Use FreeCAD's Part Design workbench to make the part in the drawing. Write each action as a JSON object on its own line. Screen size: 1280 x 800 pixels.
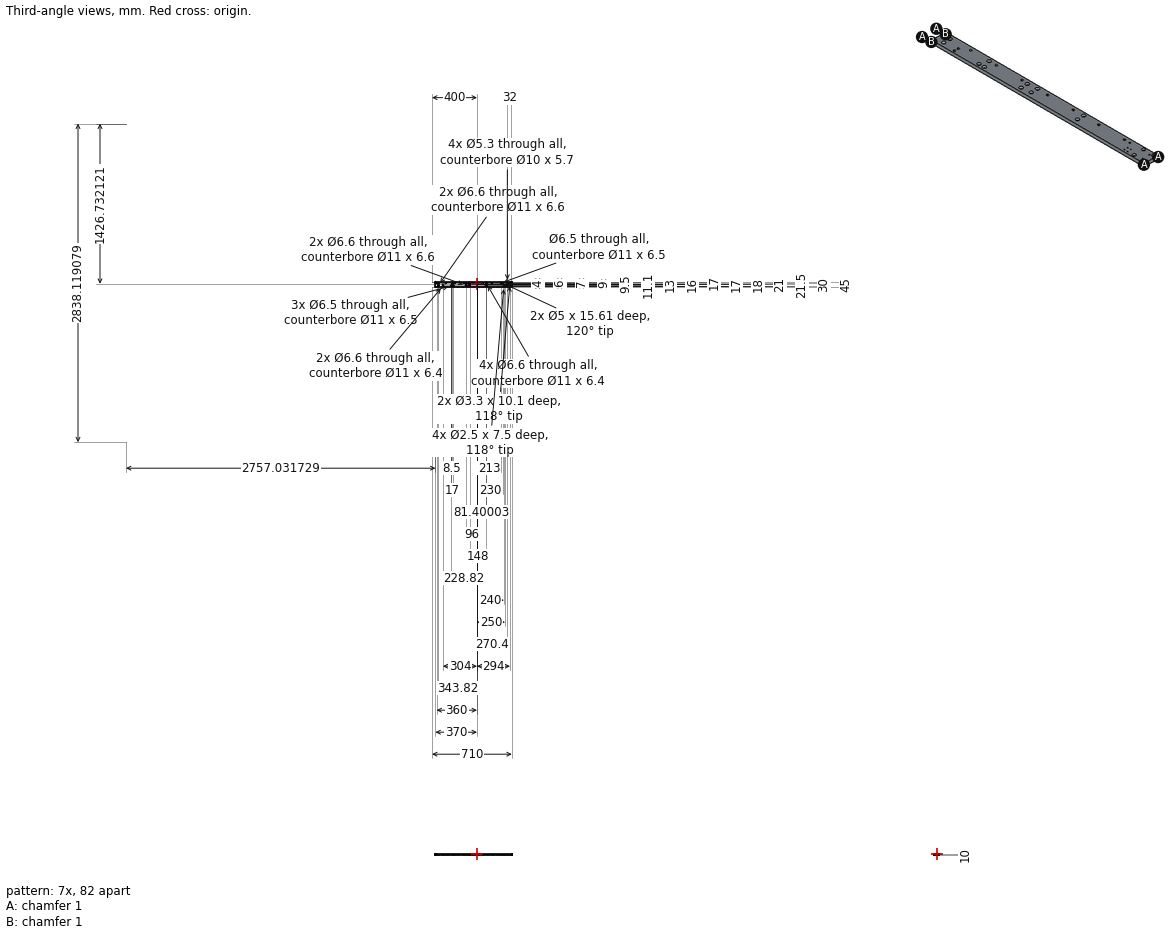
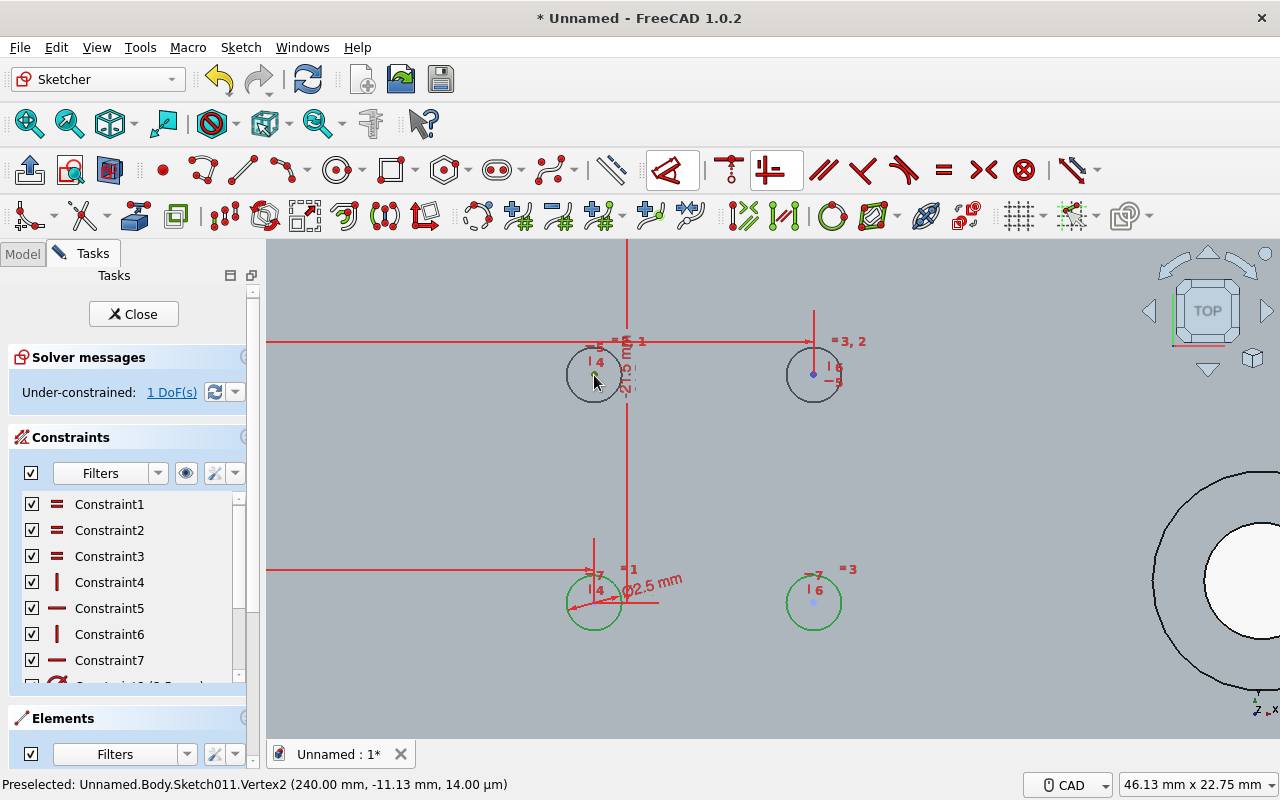
{"action": "key", "text": "i"}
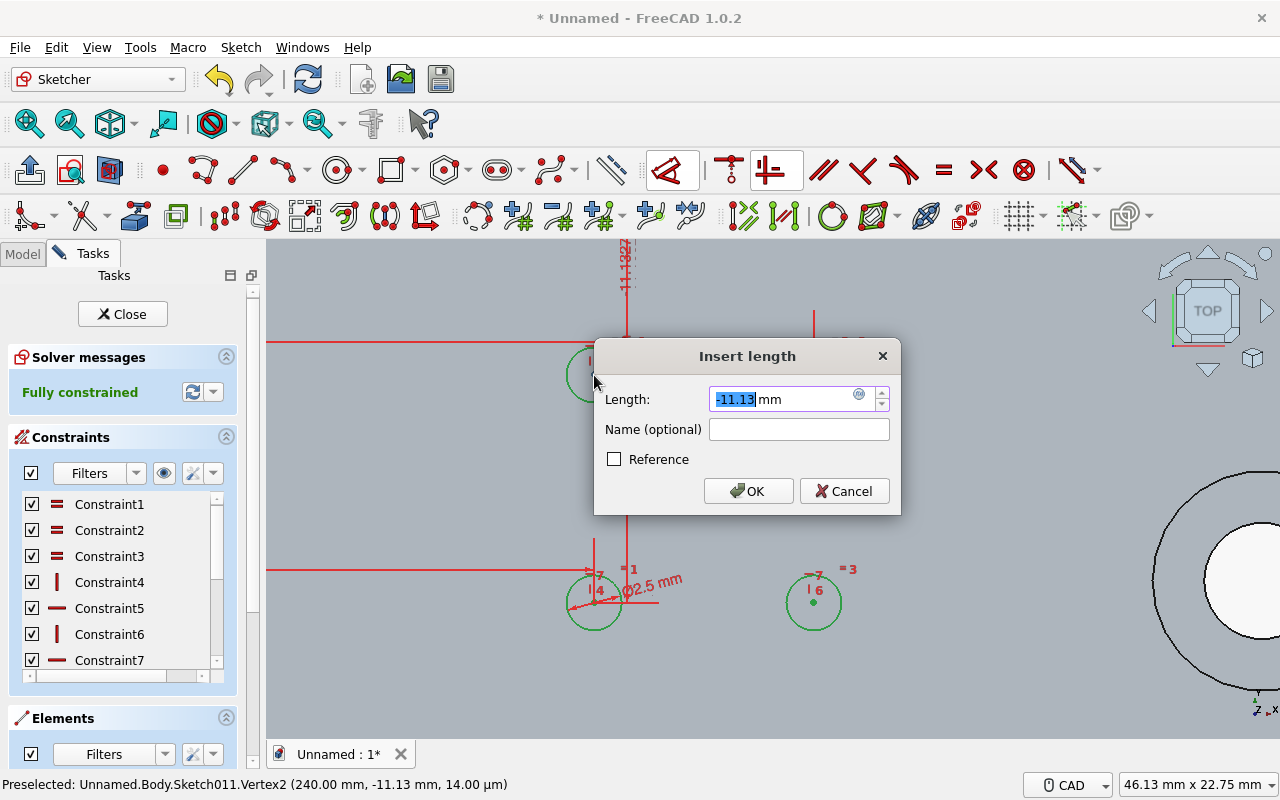
{"action": "type", "text": "-11.1"}
{"action": "key", "text": "Return"}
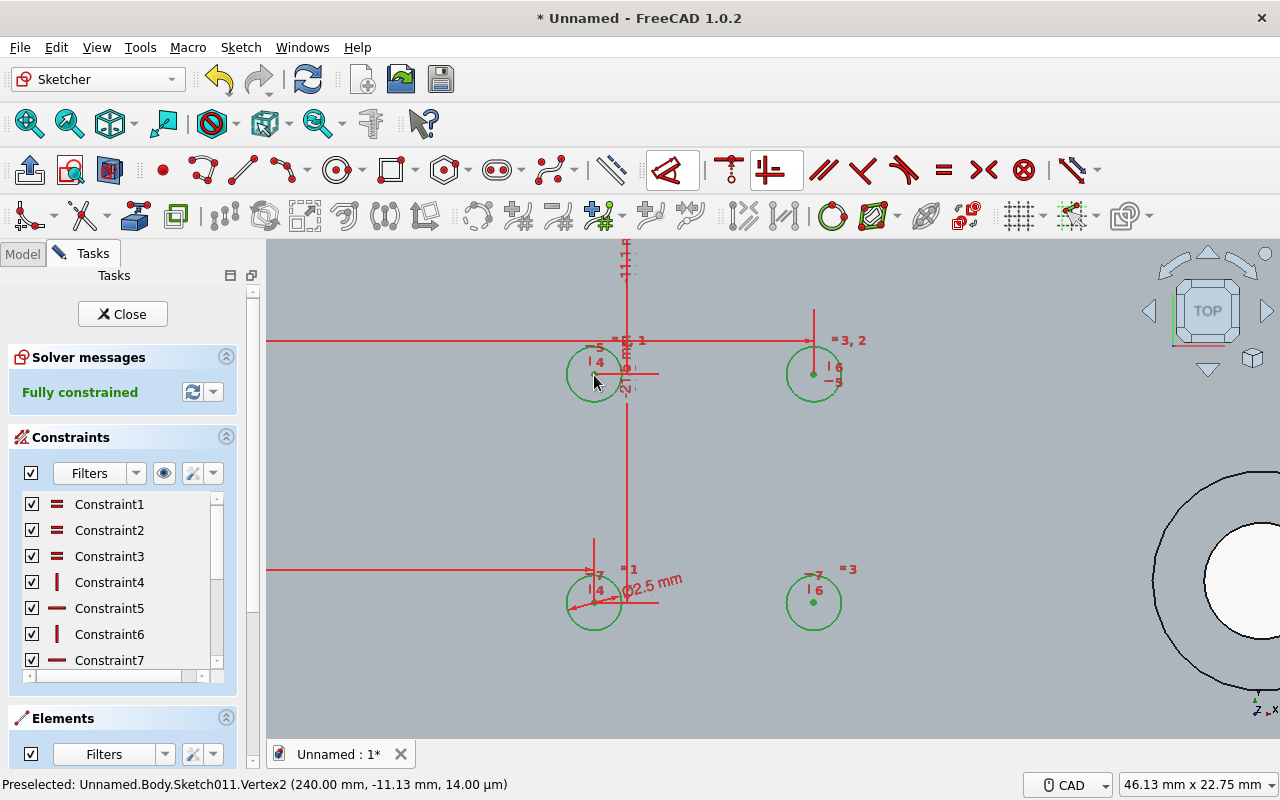
{"action": "left_click", "coordinate": [123, 314]}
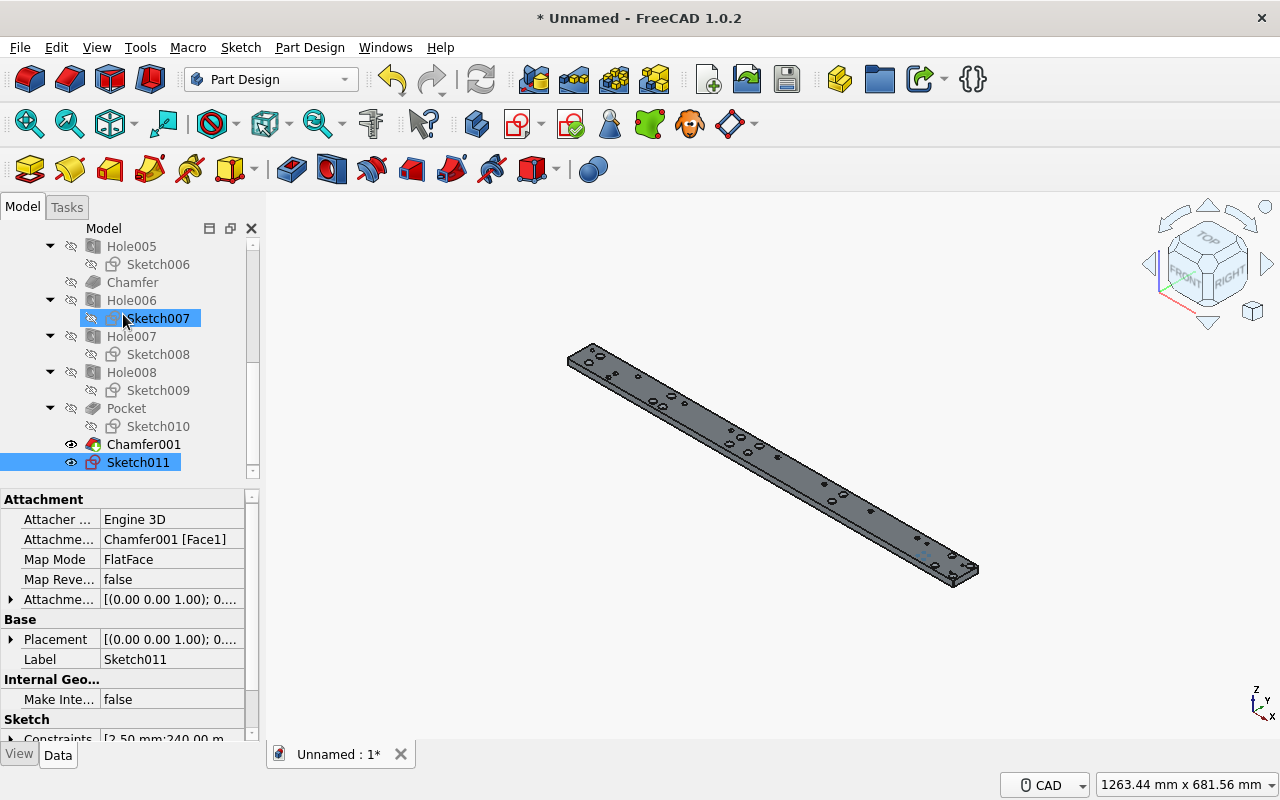
{"action": "left_click", "coordinate": [332, 170]}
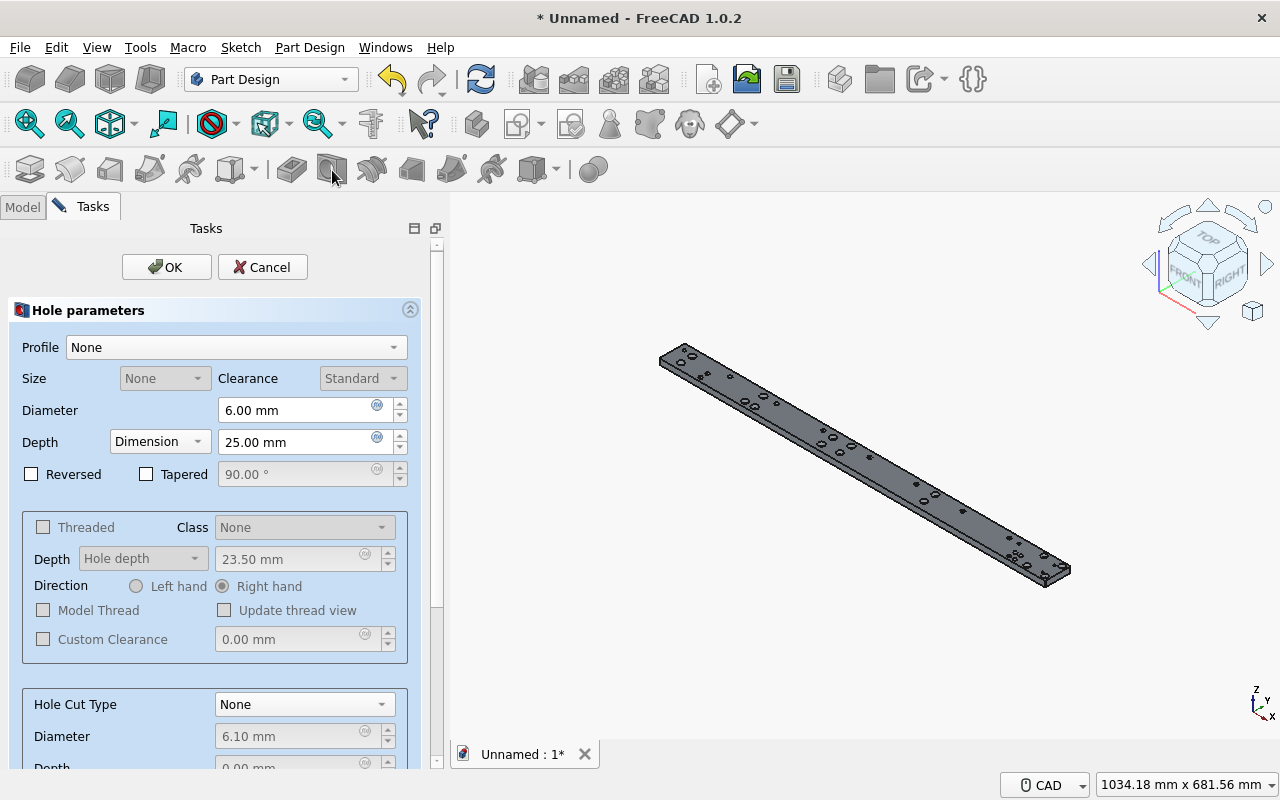
{"action": "triple_click", "coordinate": [305, 410]}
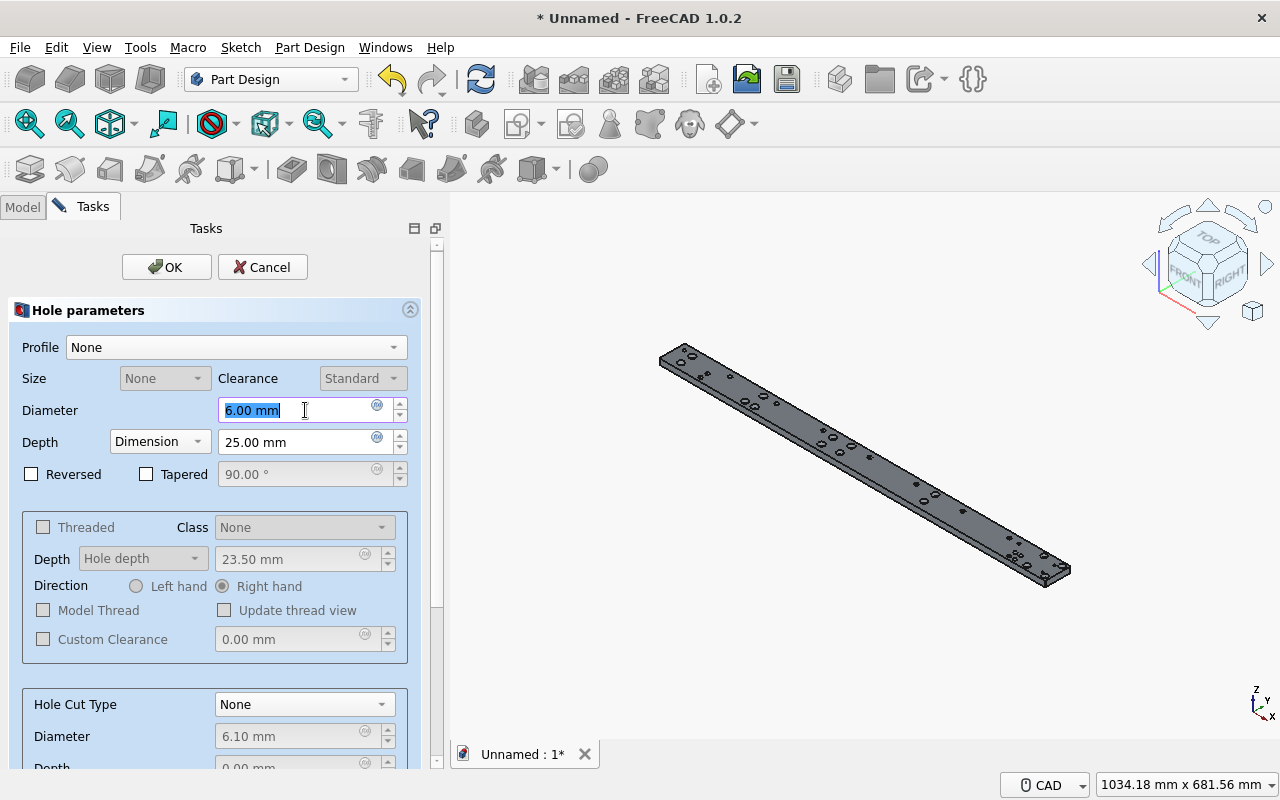
{"action": "type", "text": "2.5"}
{"action": "key", "text": "Tab"}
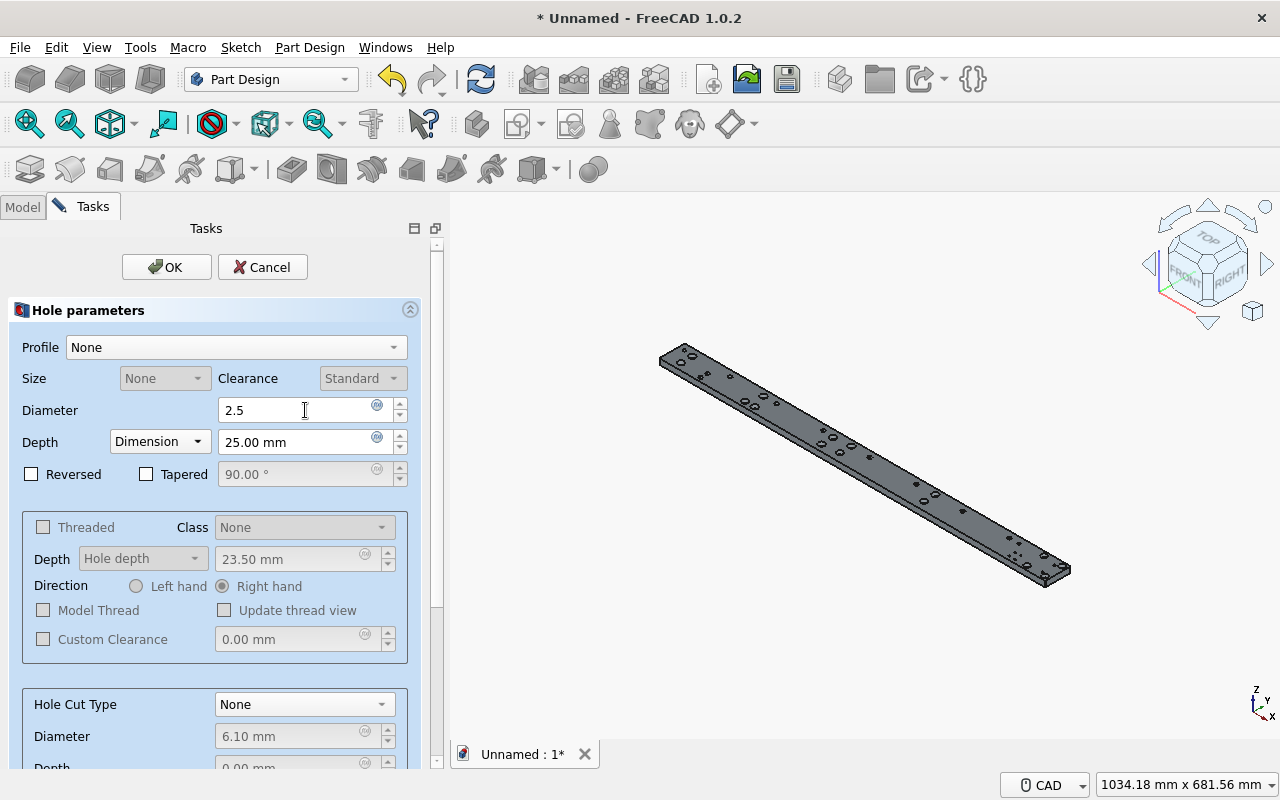
{"action": "triple_click", "coordinate": [305, 442]}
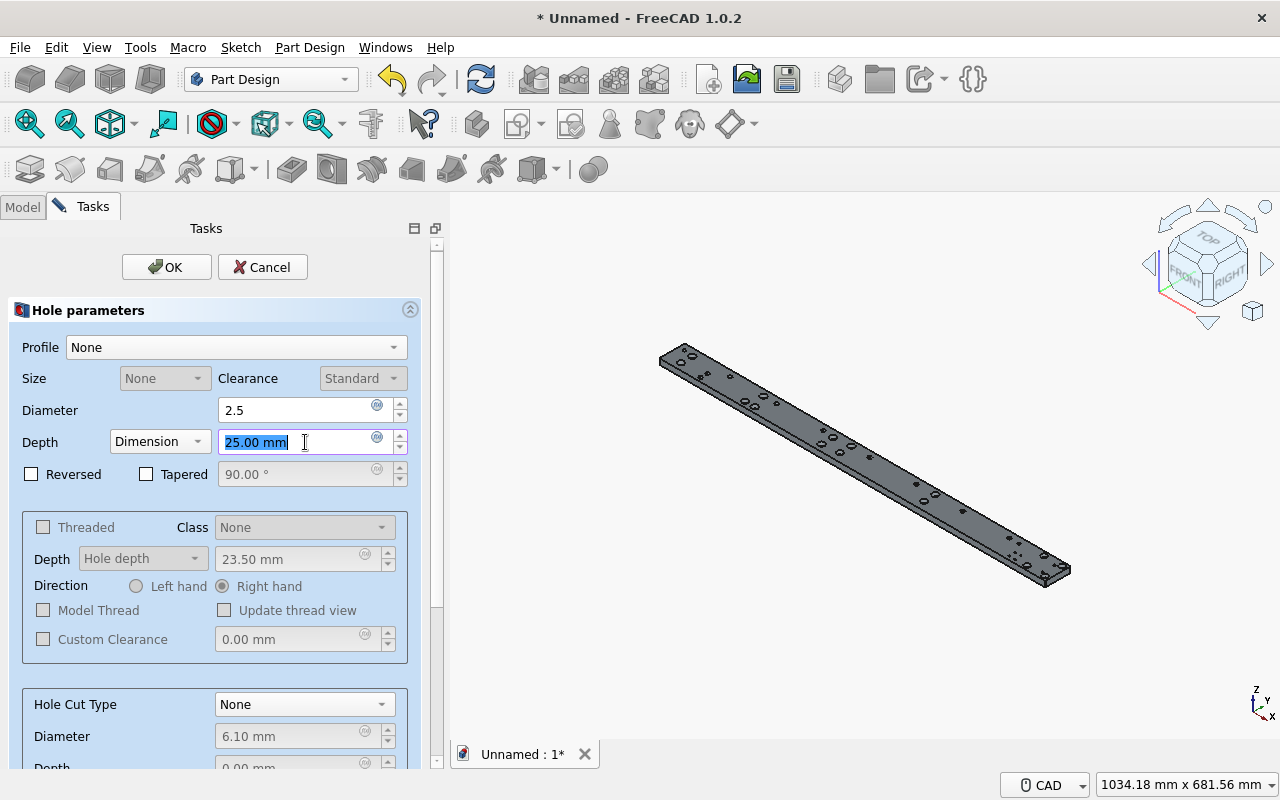
{"action": "type", "text": "7.5"}
{"action": "key", "text": "Tab"}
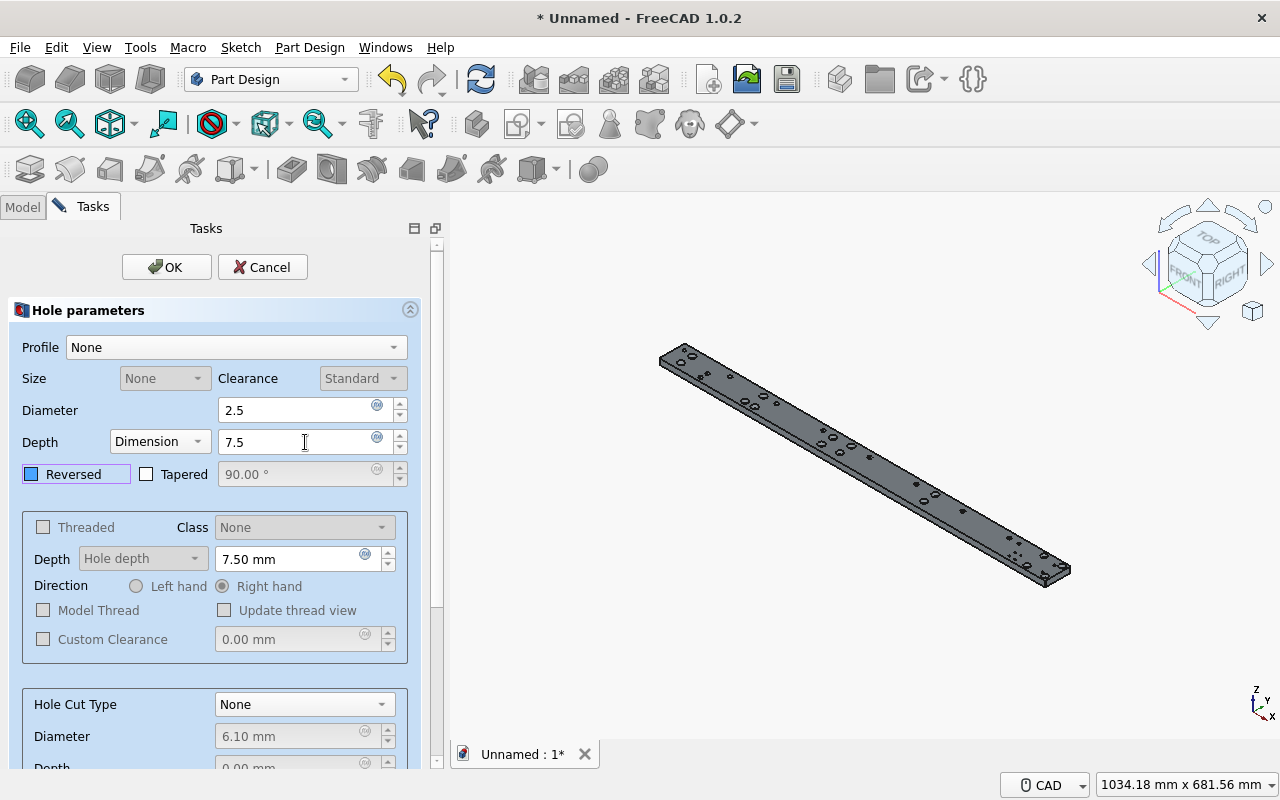
{"action": "left_click", "coordinate": [167, 267]}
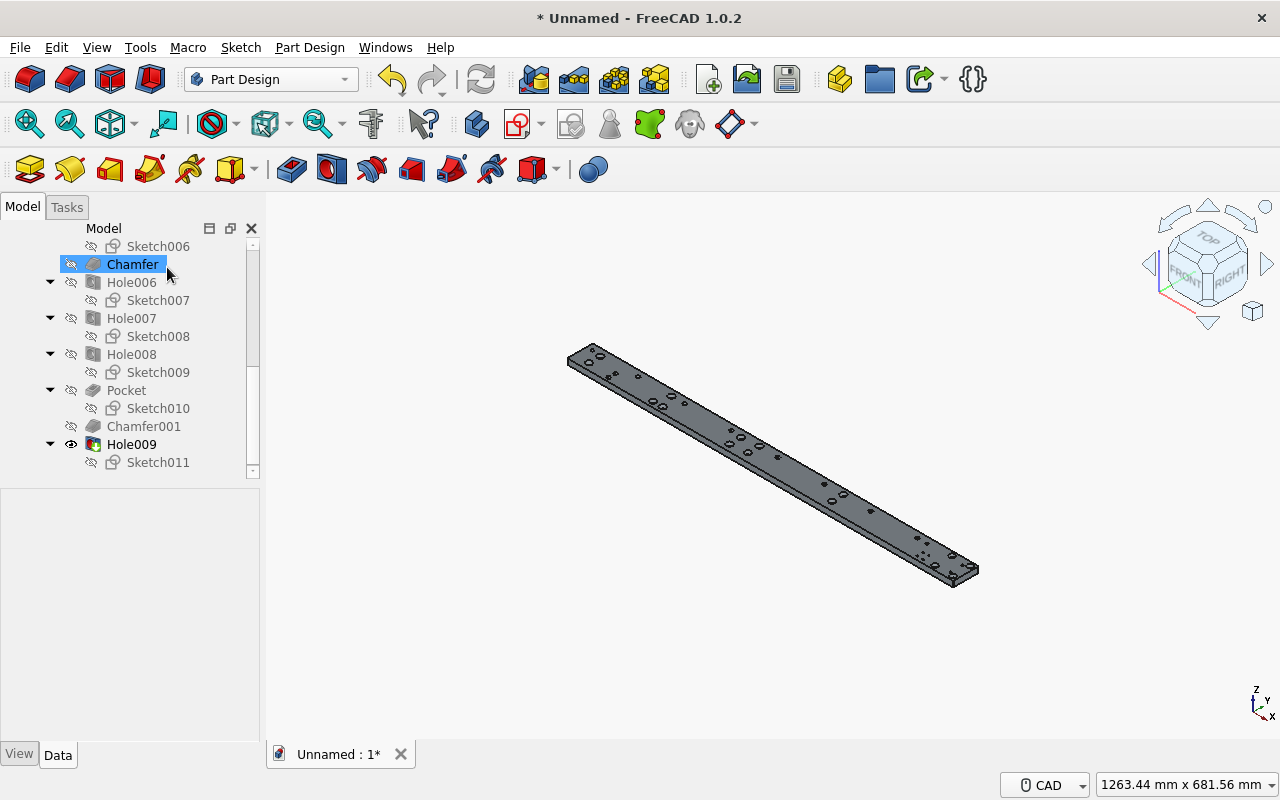
{"action": "left_click", "coordinate": [30, 124]}